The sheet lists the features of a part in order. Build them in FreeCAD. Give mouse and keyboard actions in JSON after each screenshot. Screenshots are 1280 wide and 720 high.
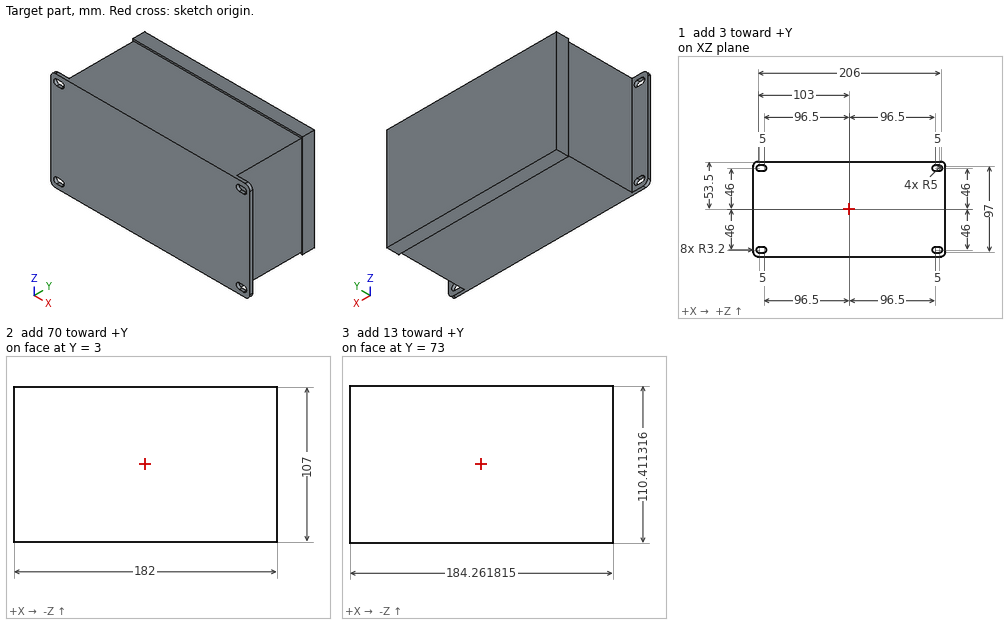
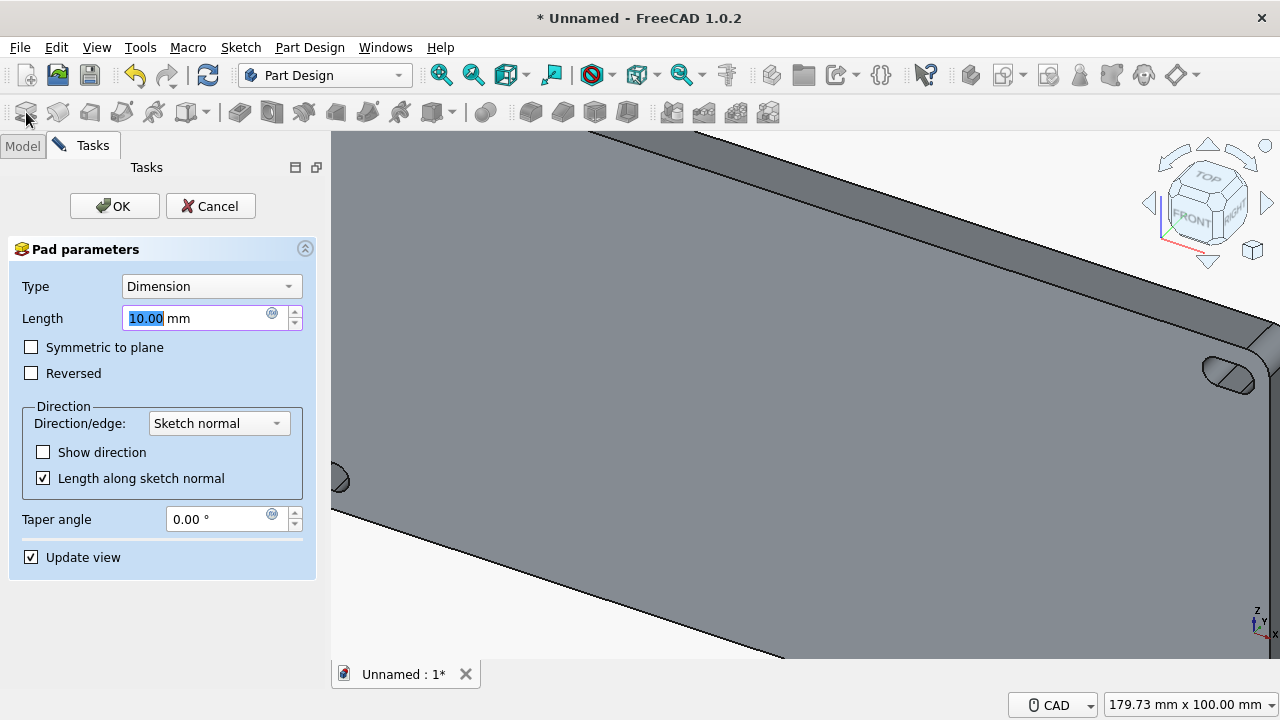
{"action": "type", "text": "3"}
{"action": "key", "text": "Tab"}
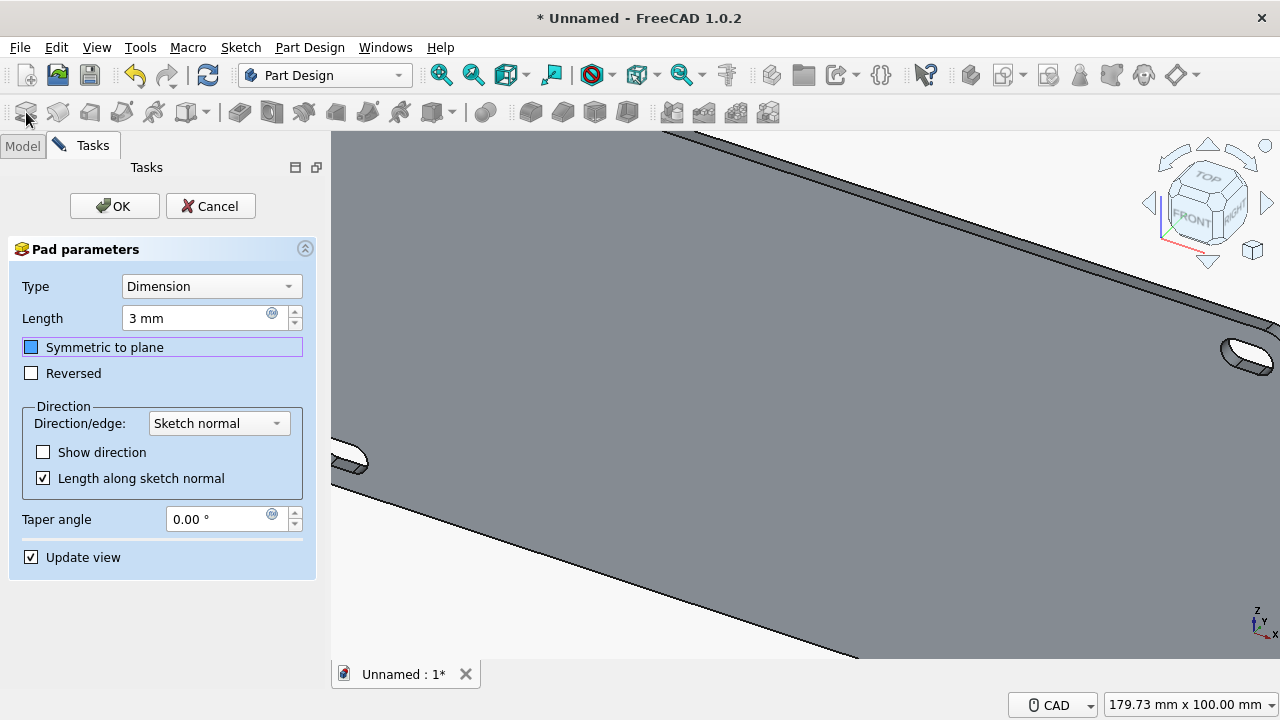
{"action": "left_click", "coordinate": [30, 373]}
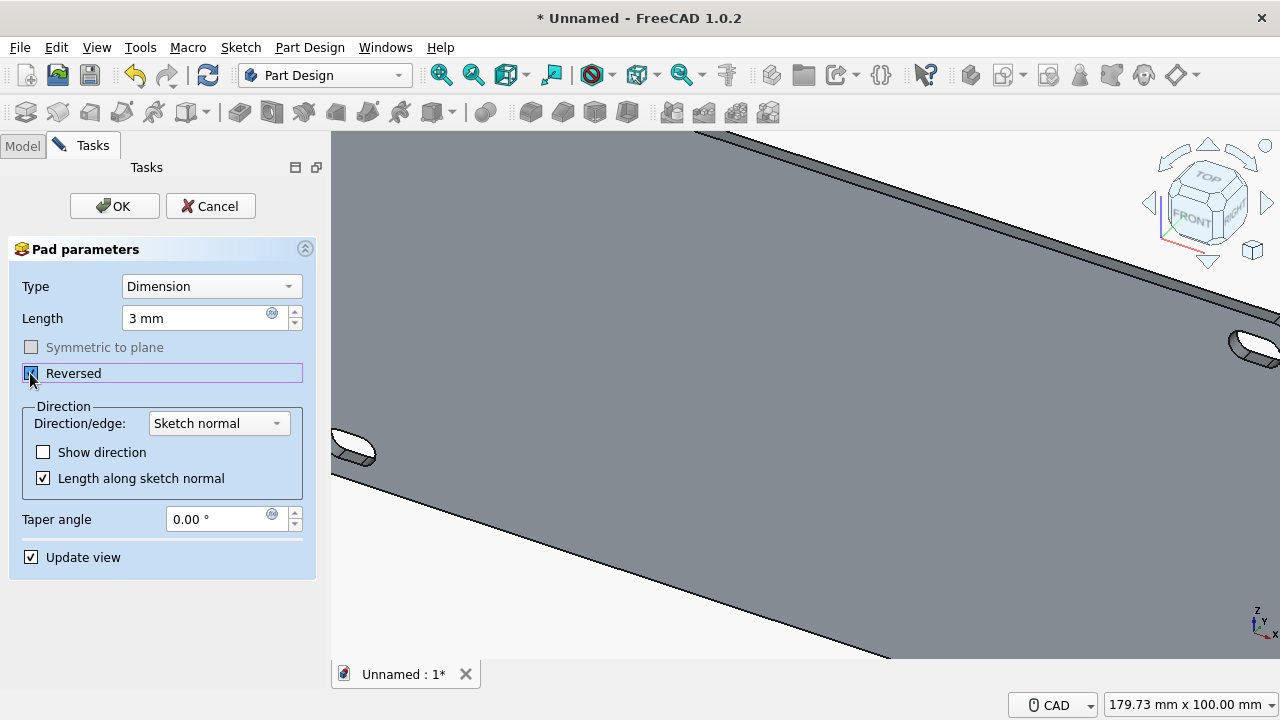
{"action": "left_click", "coordinate": [115, 206]}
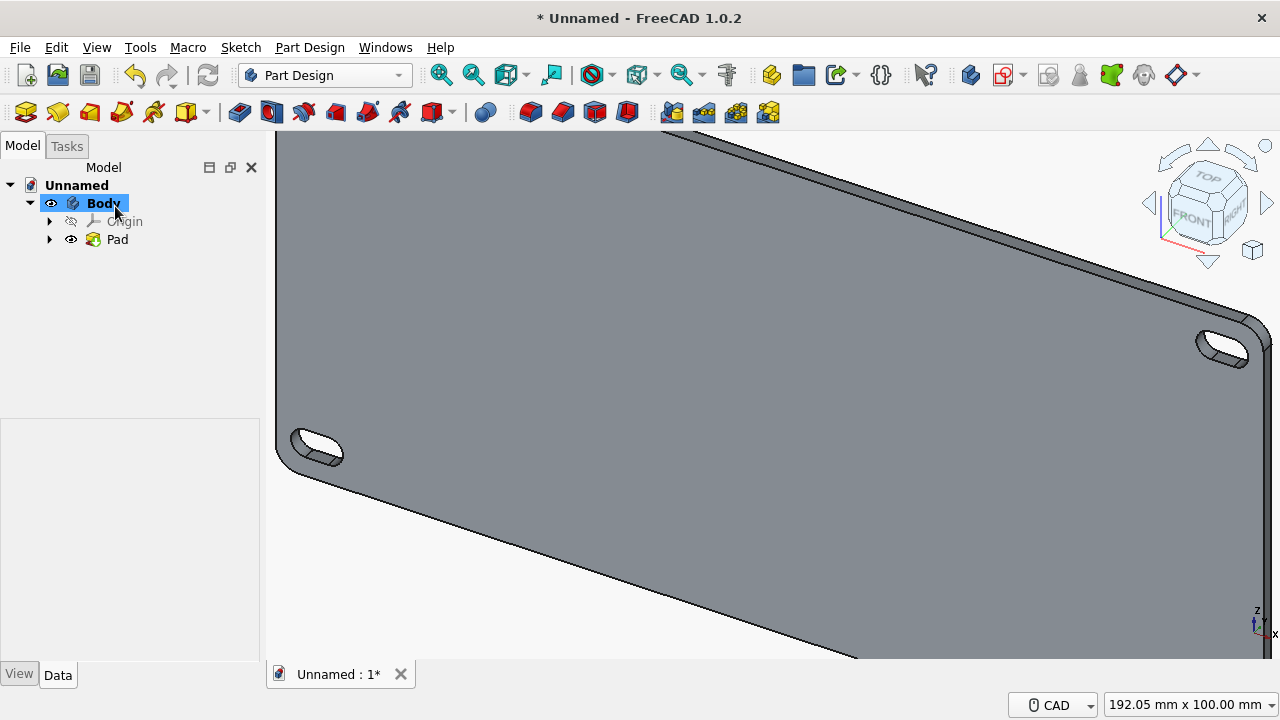
{"action": "left_click", "coordinate": [442, 76]}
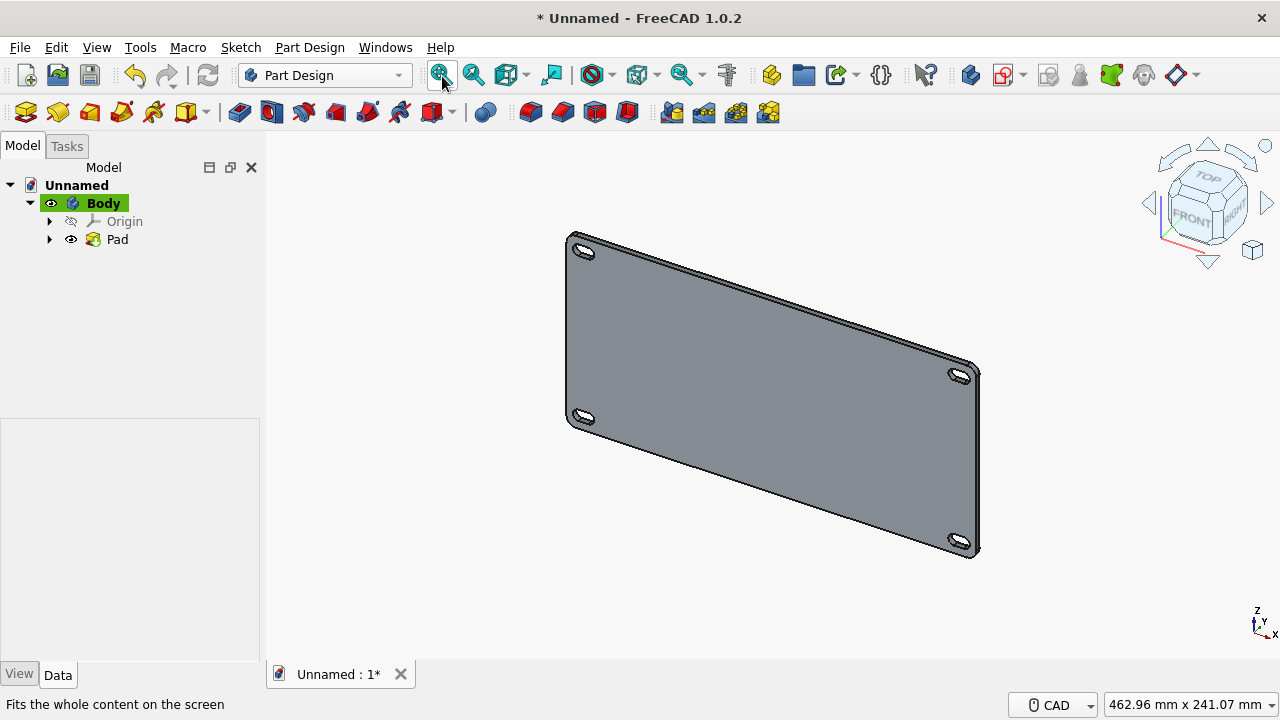
{"action": "key", "text": "4"}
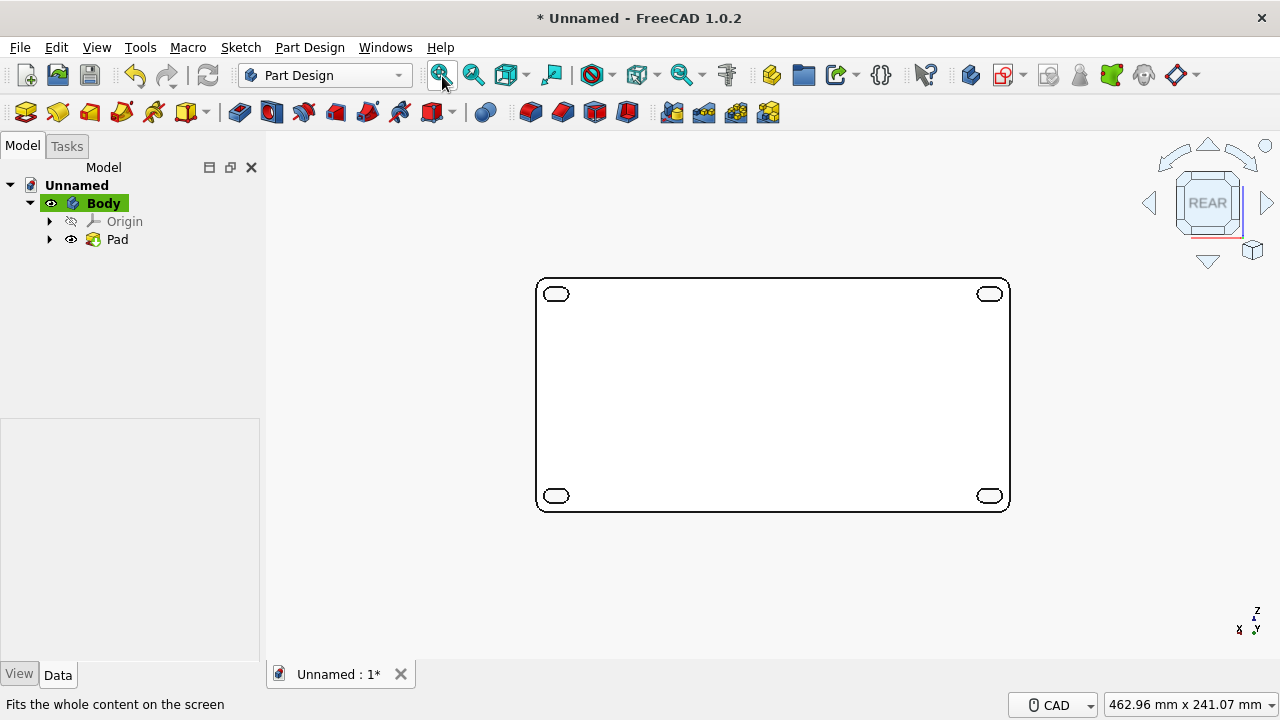
{"action": "left_click", "coordinate": [705, 394]}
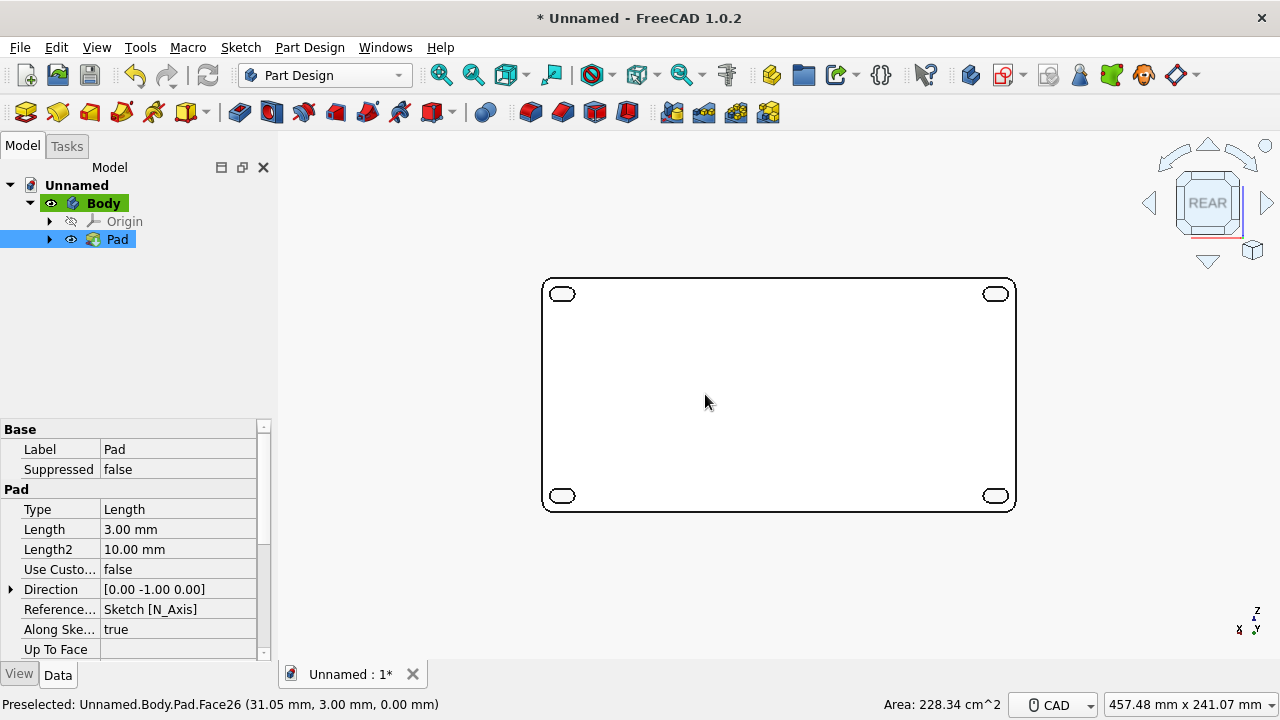
{"action": "left_click", "coordinate": [1004, 76]}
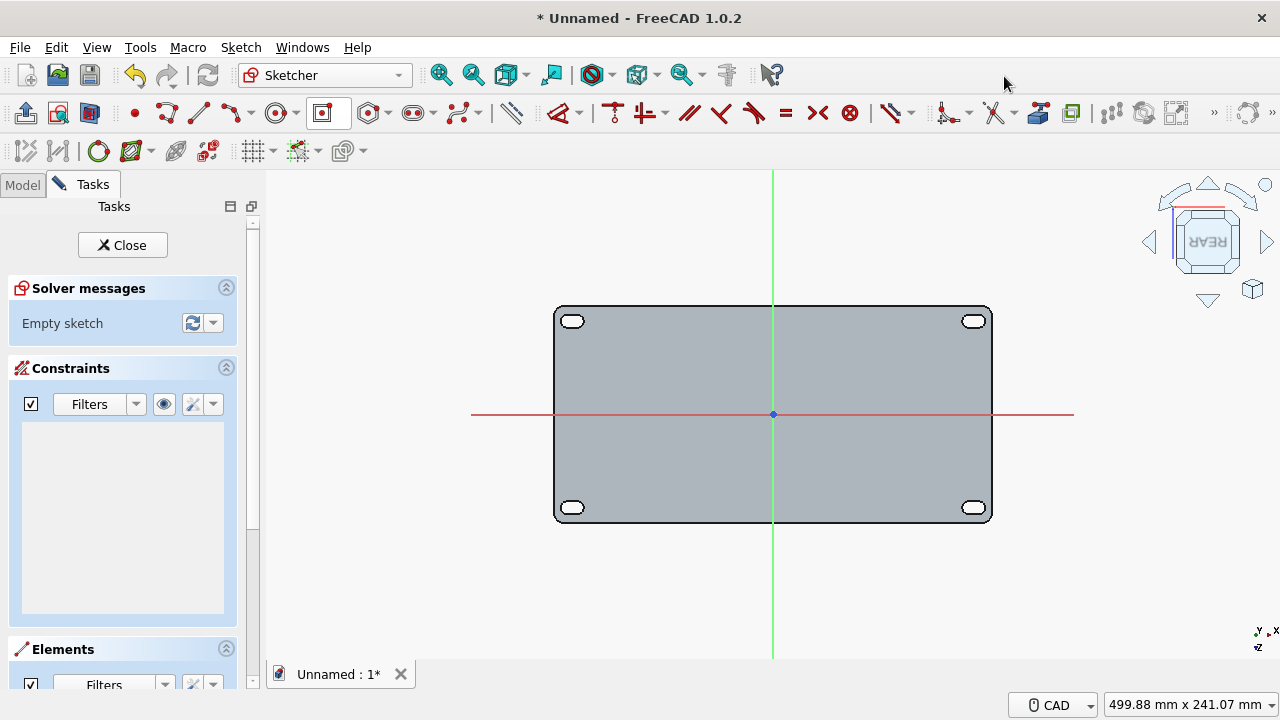
{"action": "scroll", "coordinate": [912, 415], "scroll_direction": "up", "scroll_amount": 2}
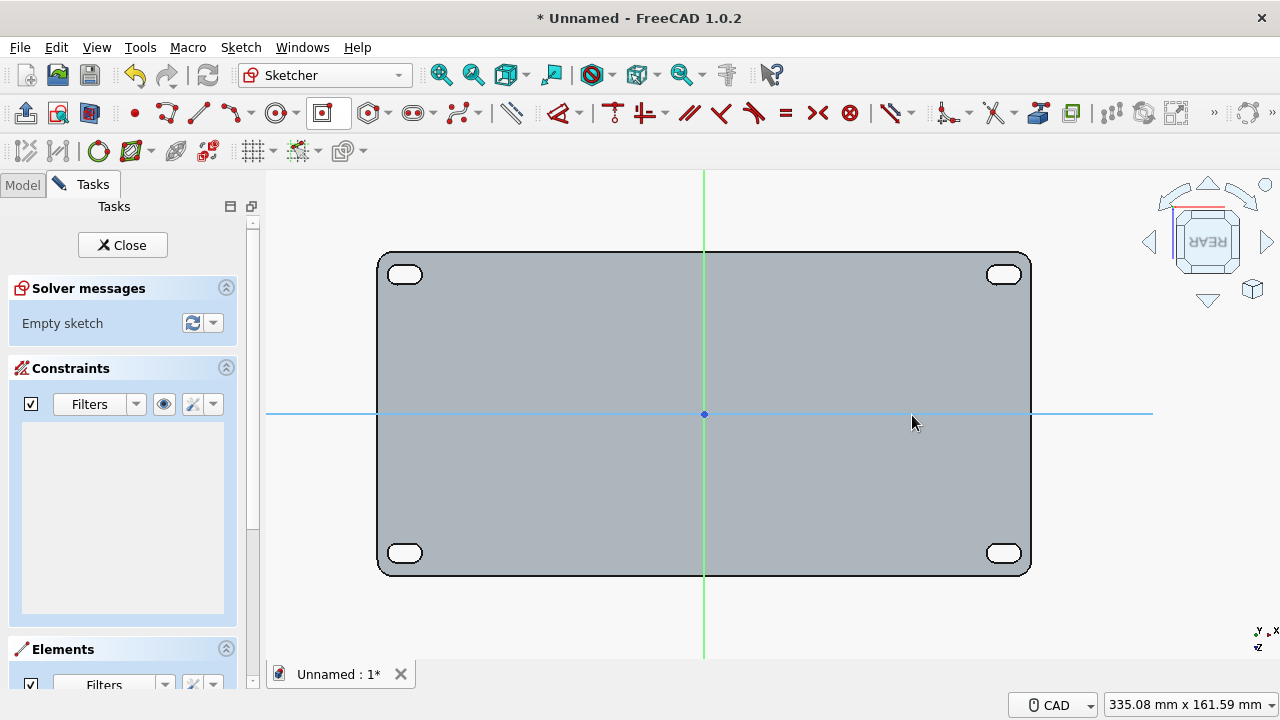
{"action": "key", "text": "g v"}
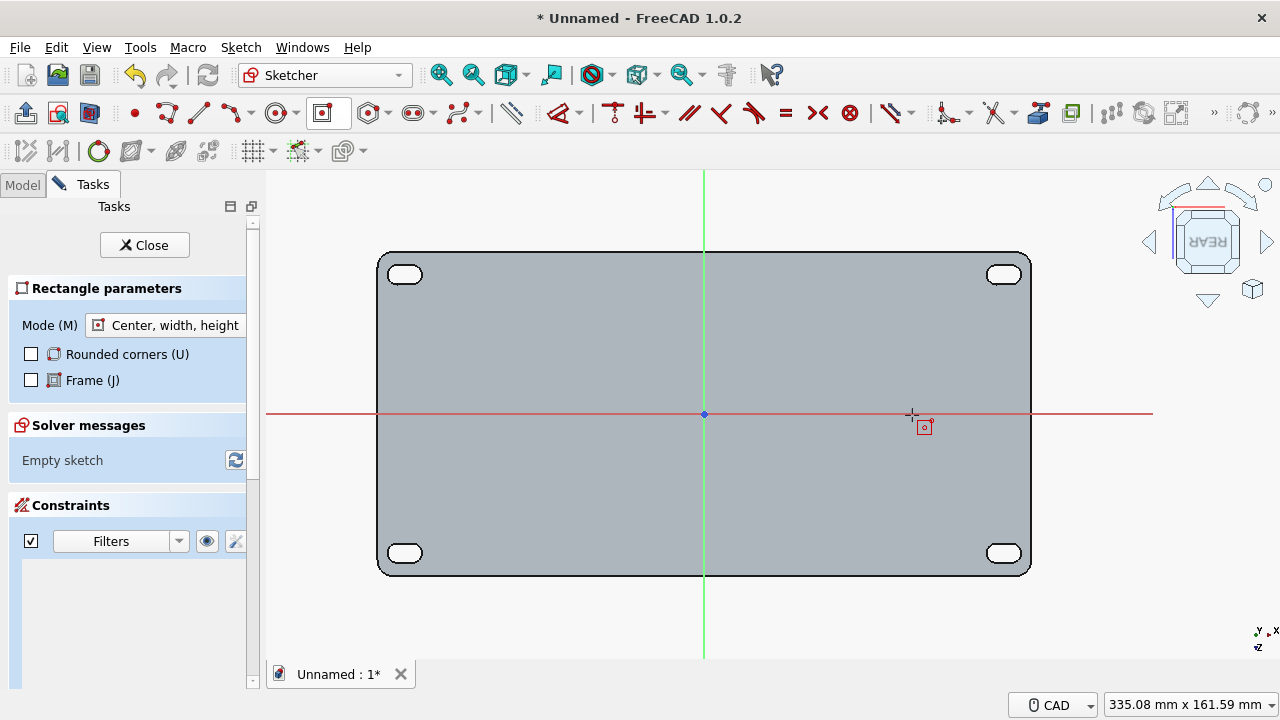
{"action": "left_click", "coordinate": [704, 414]}
{"action": "left_click", "coordinate": [980, 252]}
{"action": "key", "text": "Escape"}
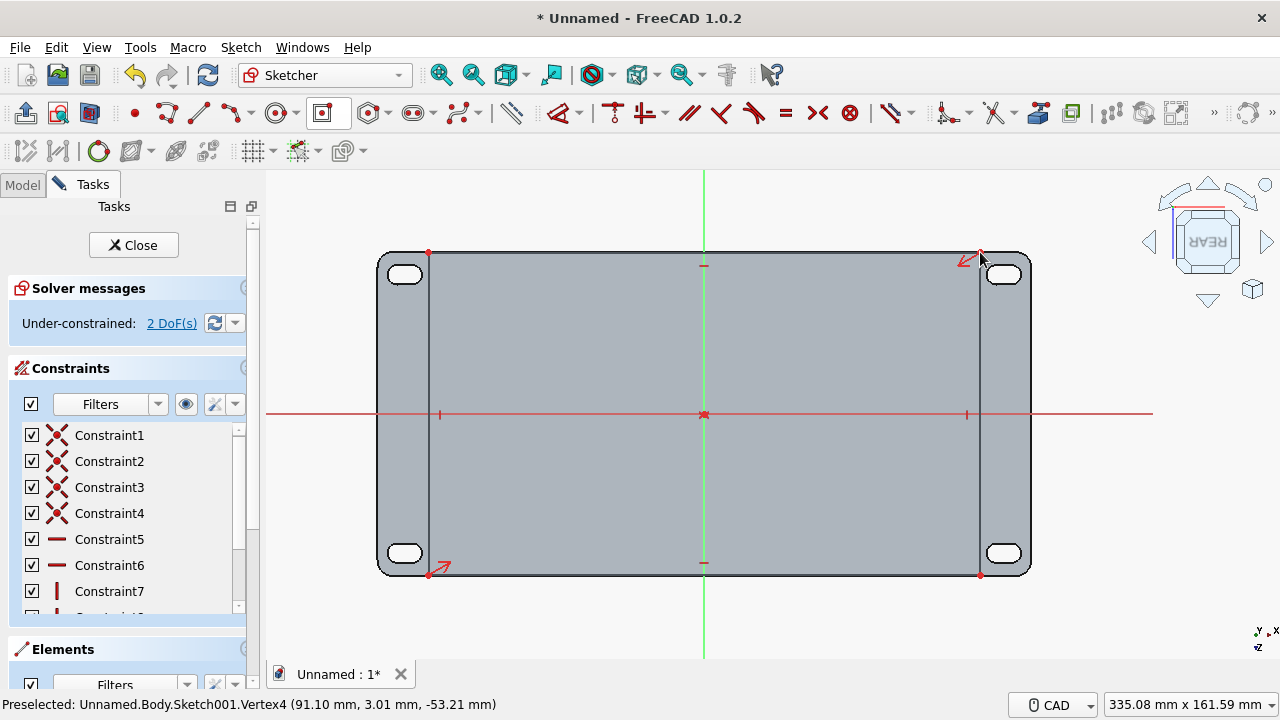
{"action": "left_click", "coordinate": [558, 114]}